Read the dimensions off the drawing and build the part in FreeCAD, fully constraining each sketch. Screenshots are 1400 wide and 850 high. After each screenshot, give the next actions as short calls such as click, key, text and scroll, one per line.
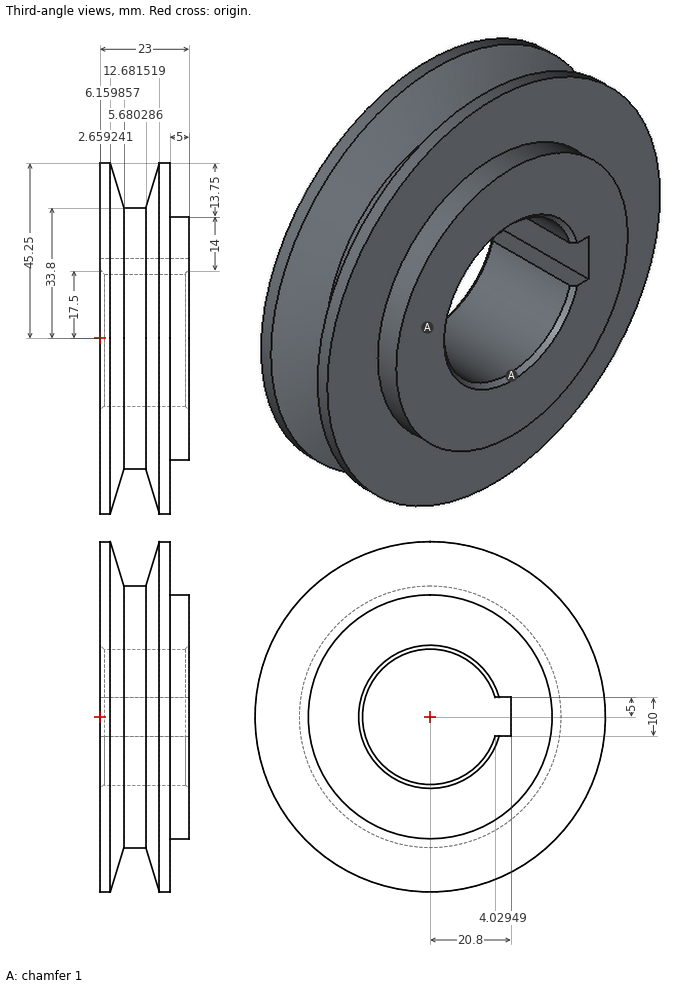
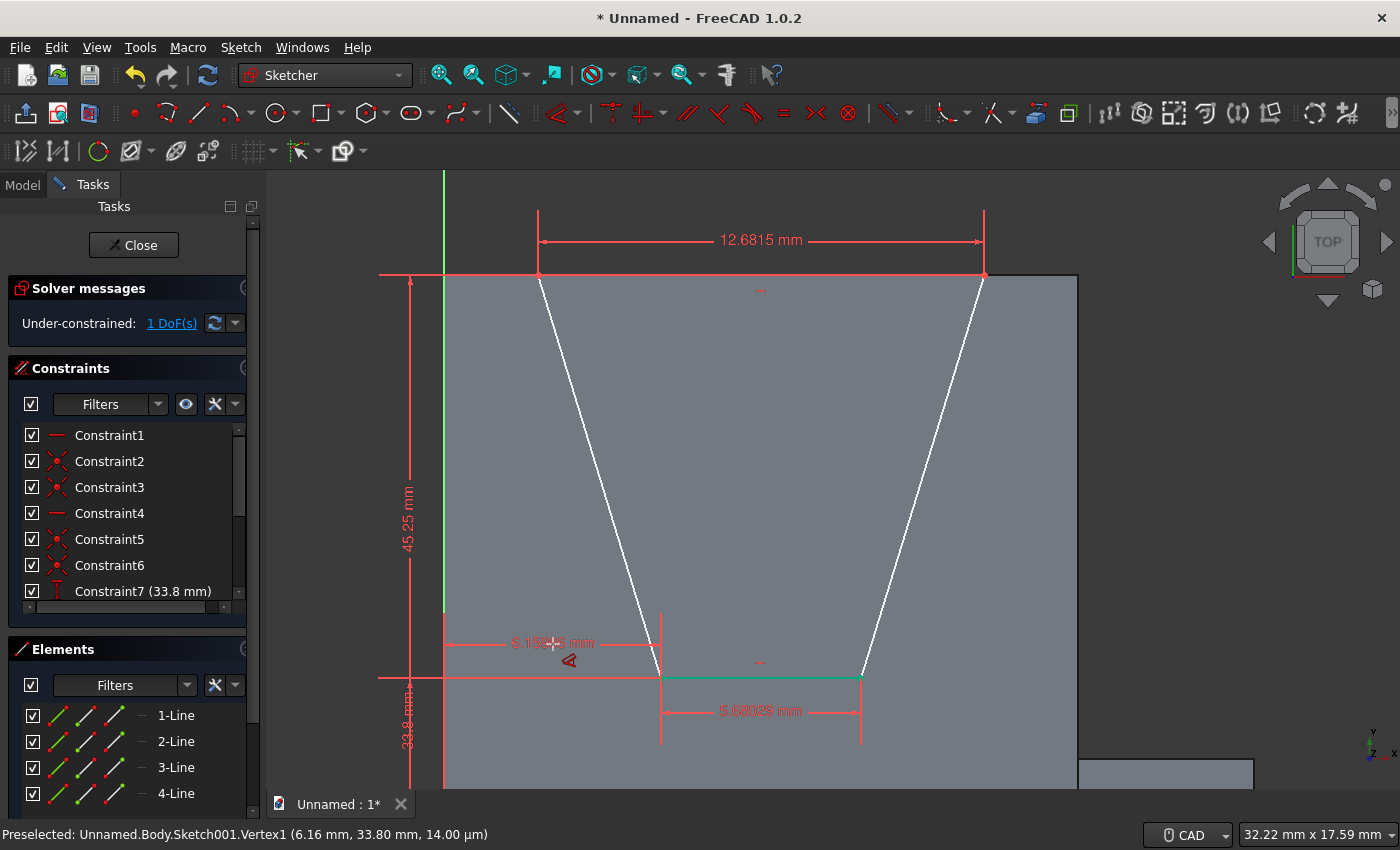
click(538, 275)
click(491, 241)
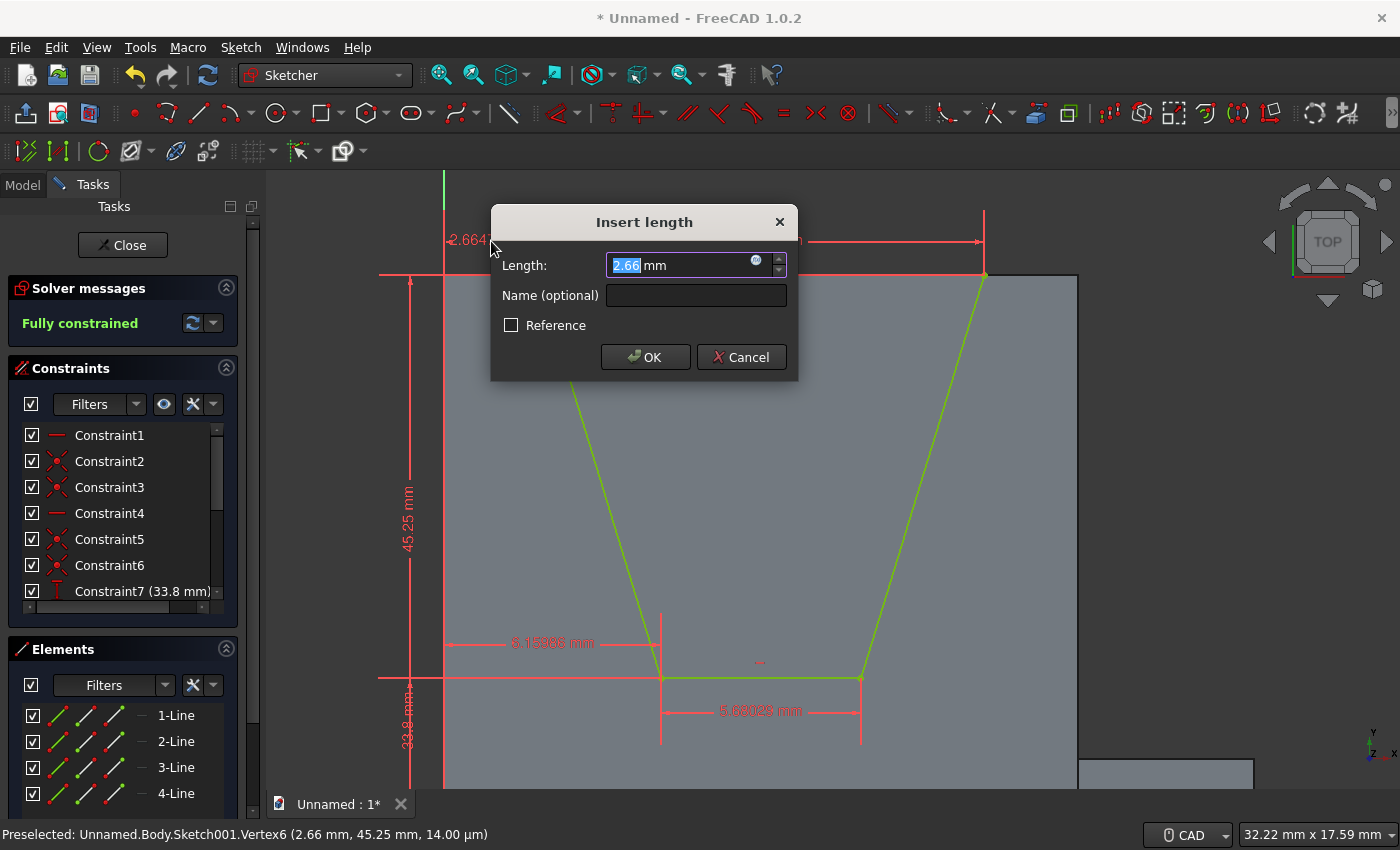
text(2.659241)
key(Return)
key(Escape)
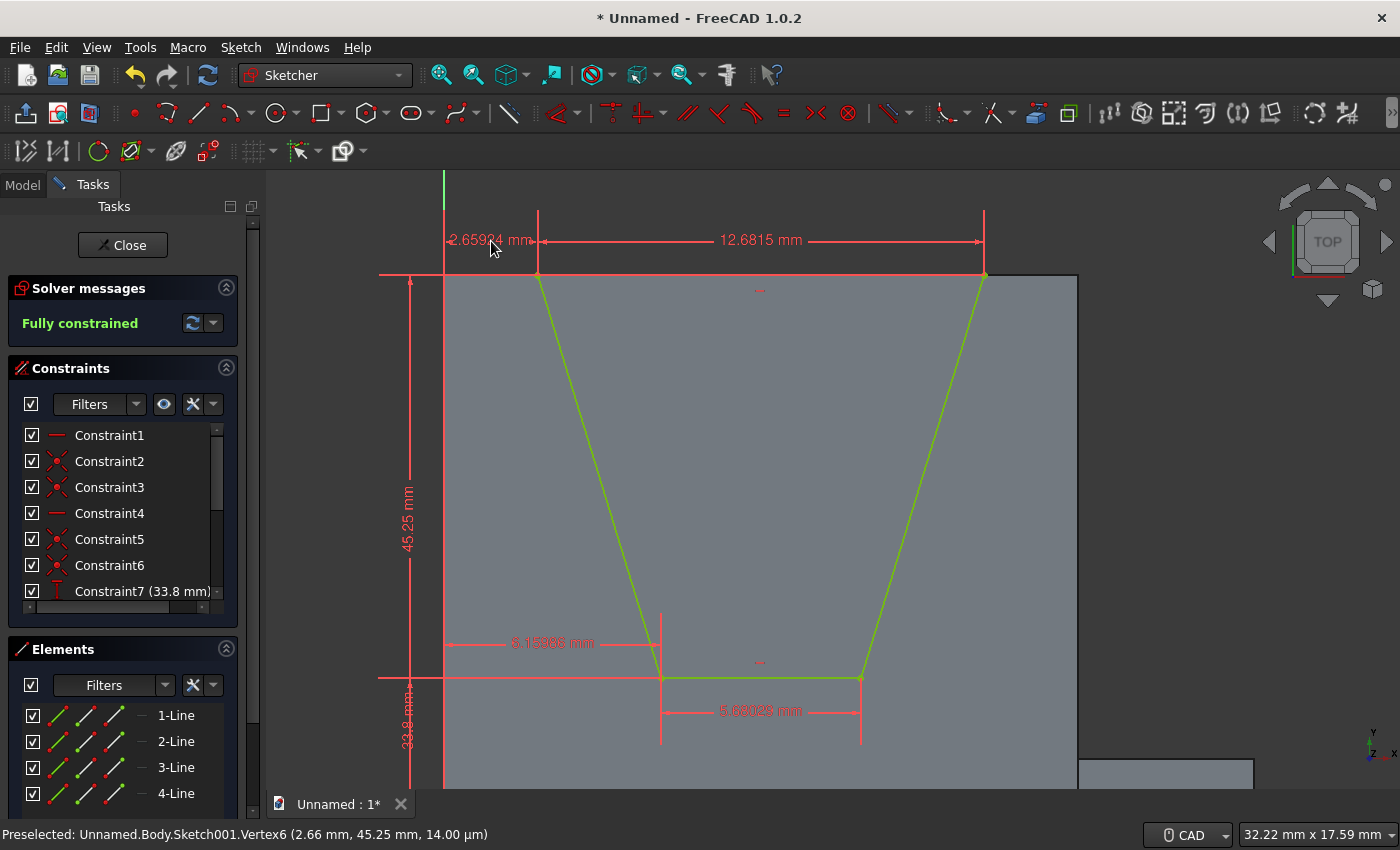
click(123, 245)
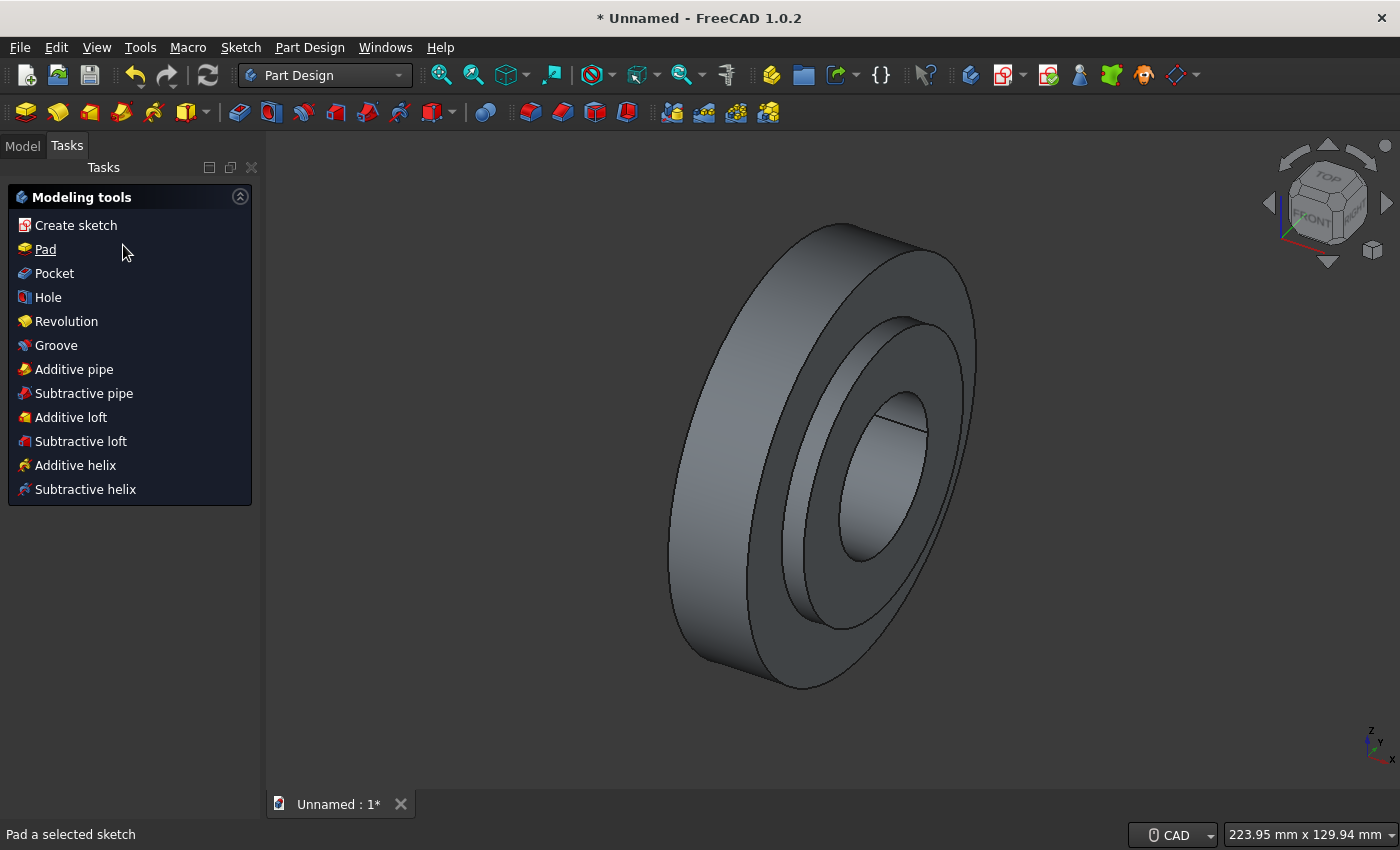
click(304, 112)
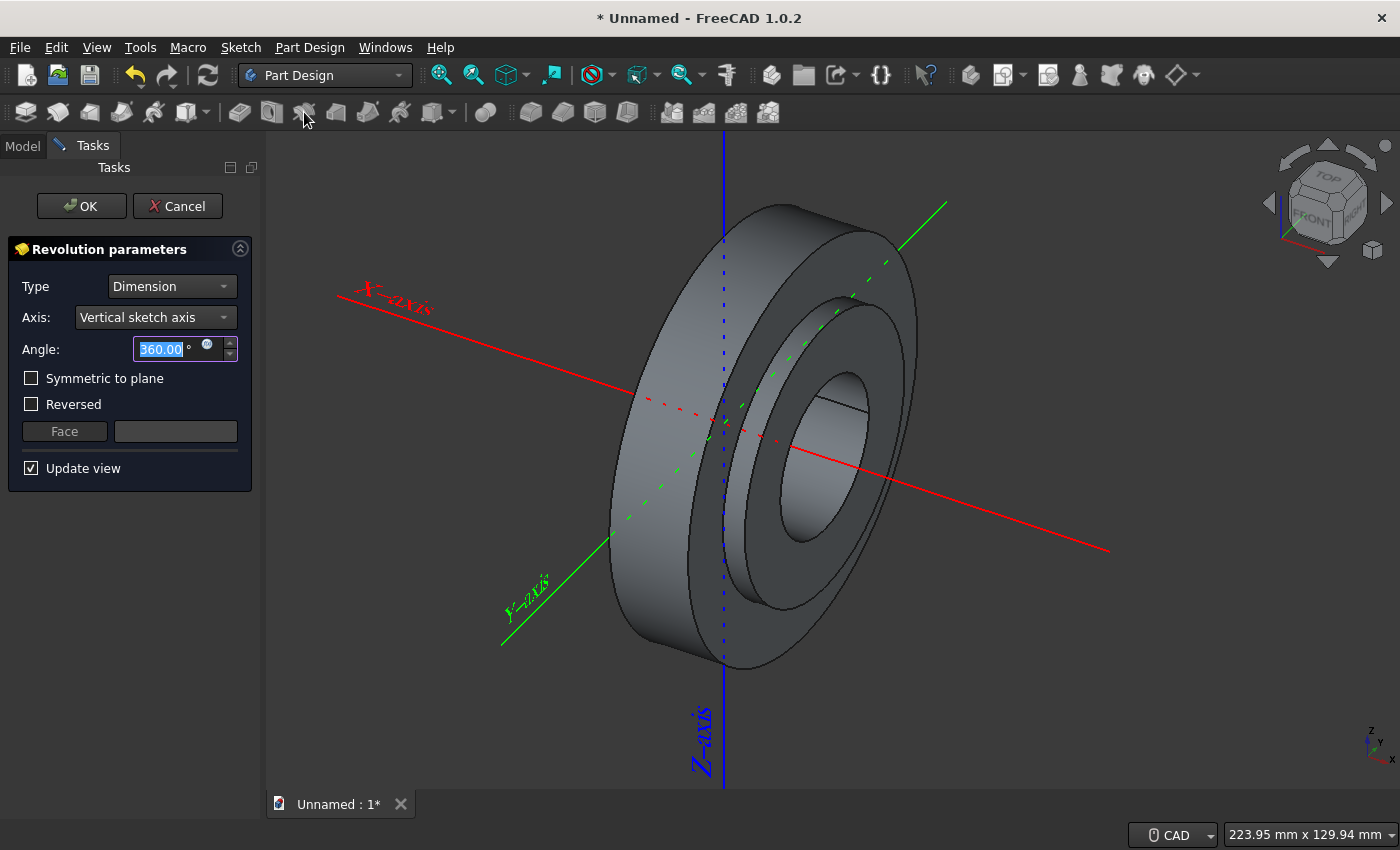
click(156, 318)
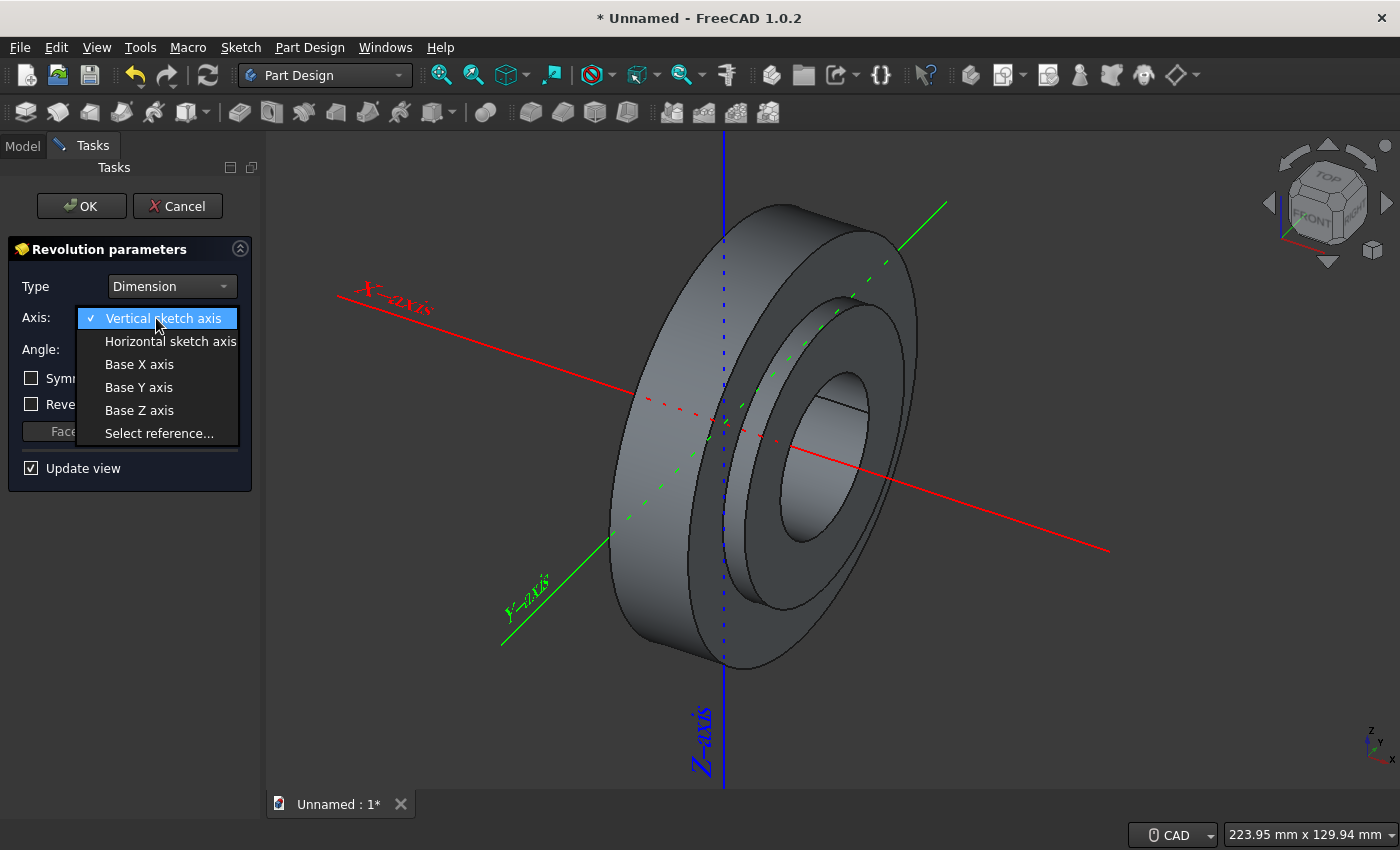
click(156, 342)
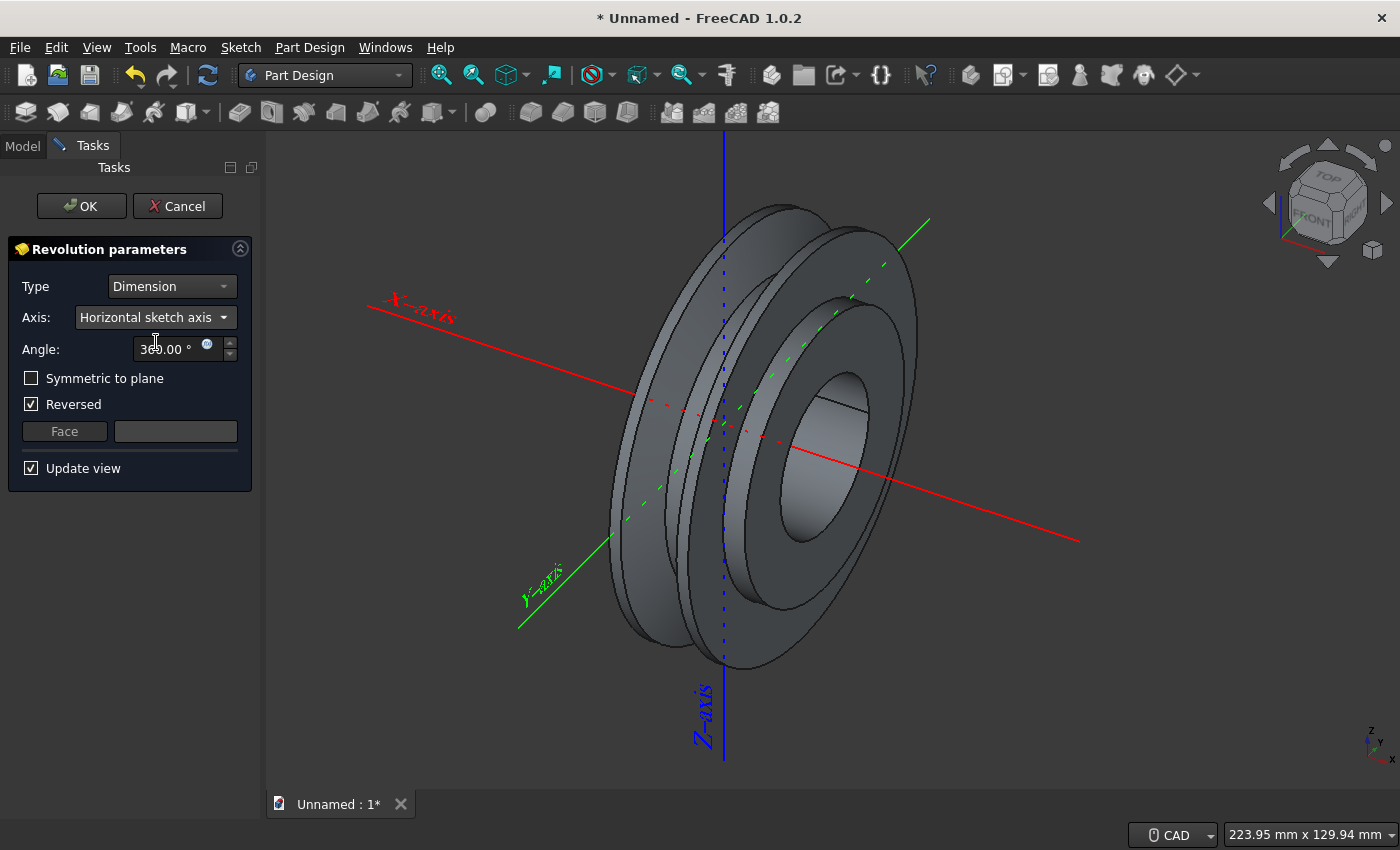
click(82, 206)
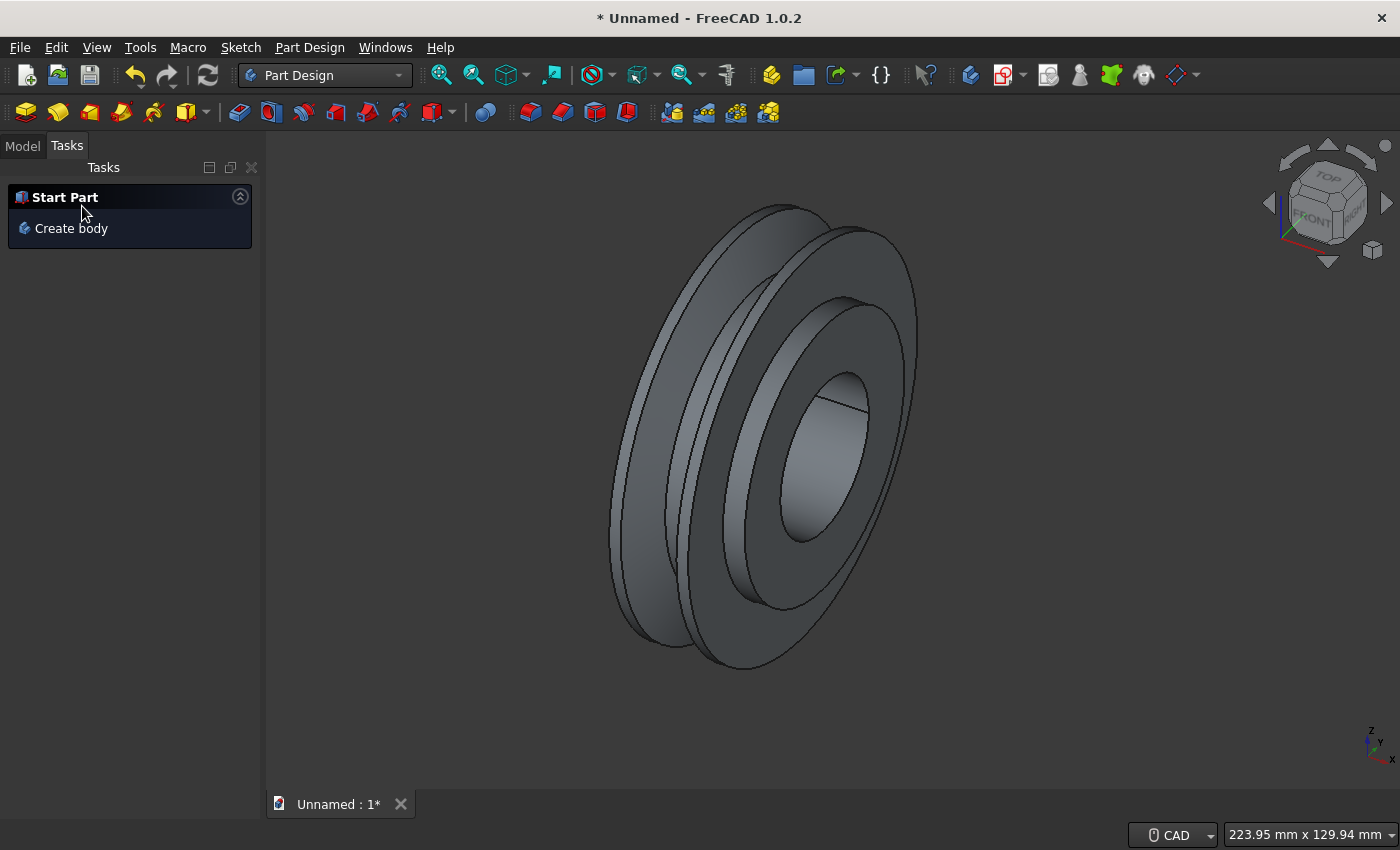
key(v)
key(f)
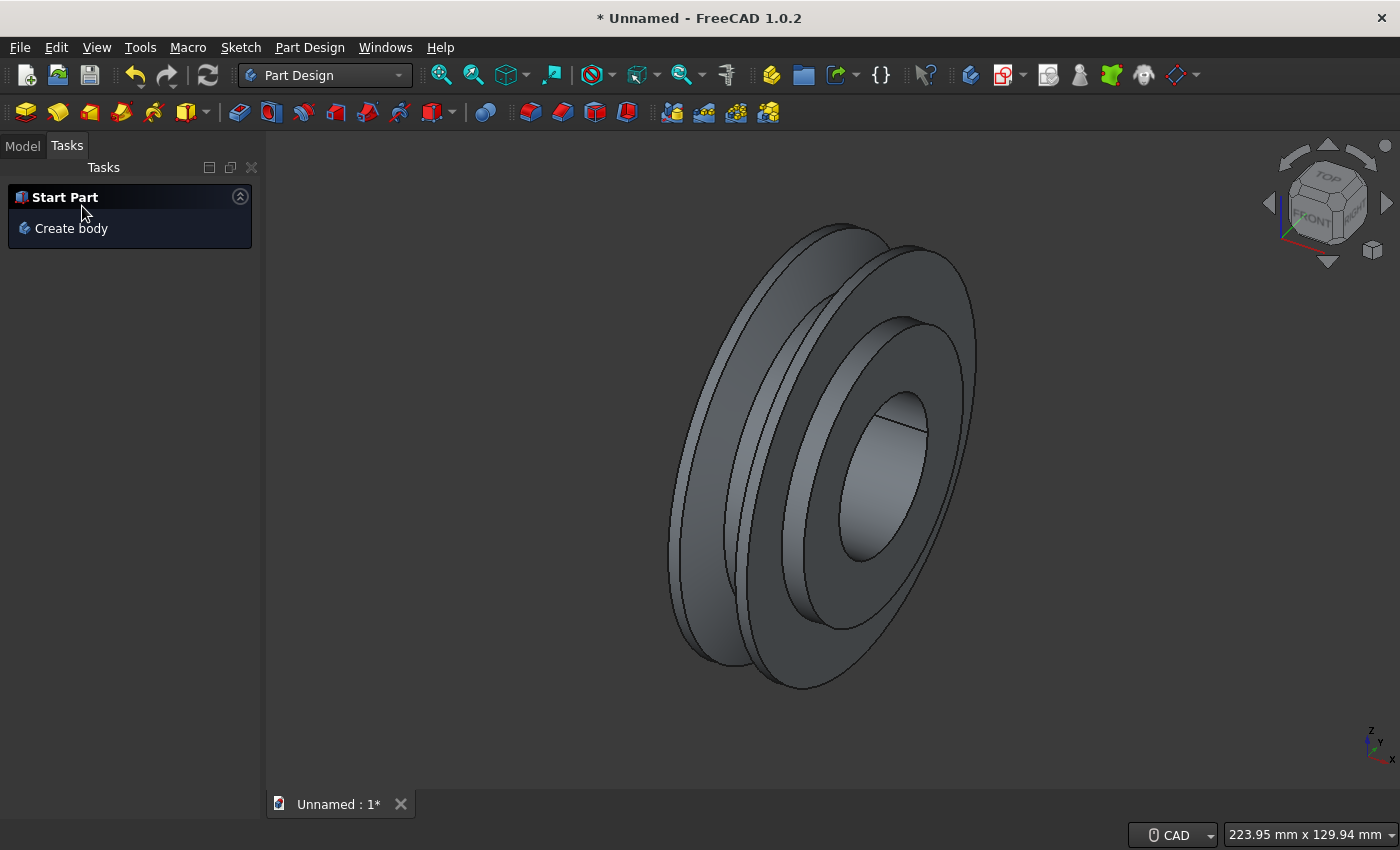
click(870, 558)